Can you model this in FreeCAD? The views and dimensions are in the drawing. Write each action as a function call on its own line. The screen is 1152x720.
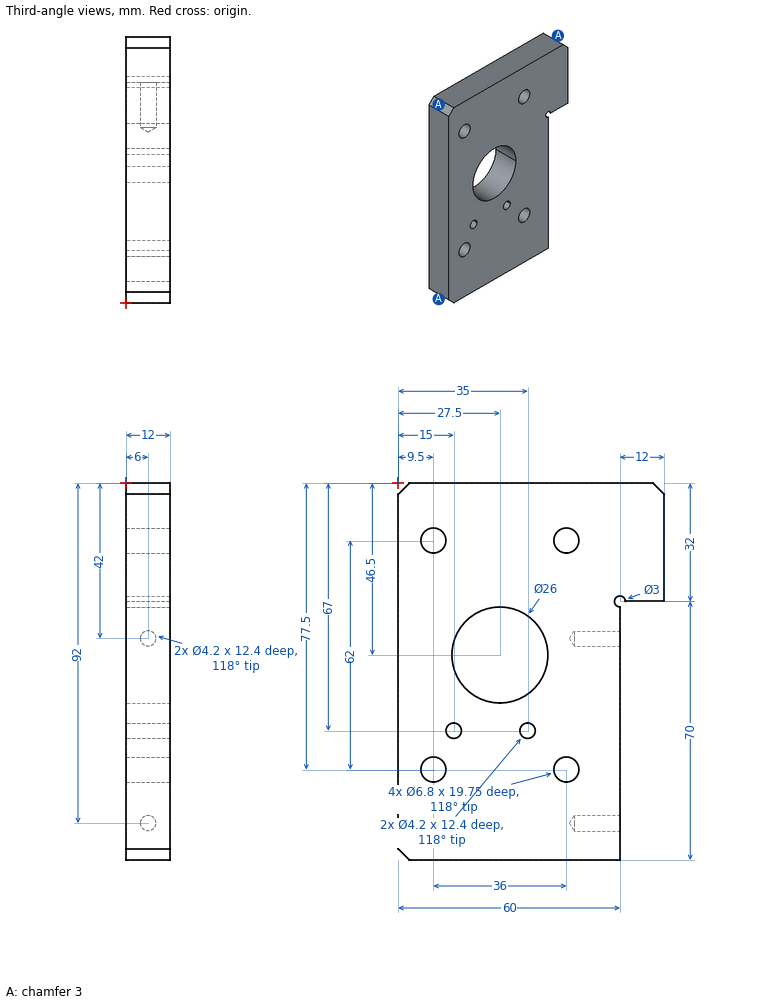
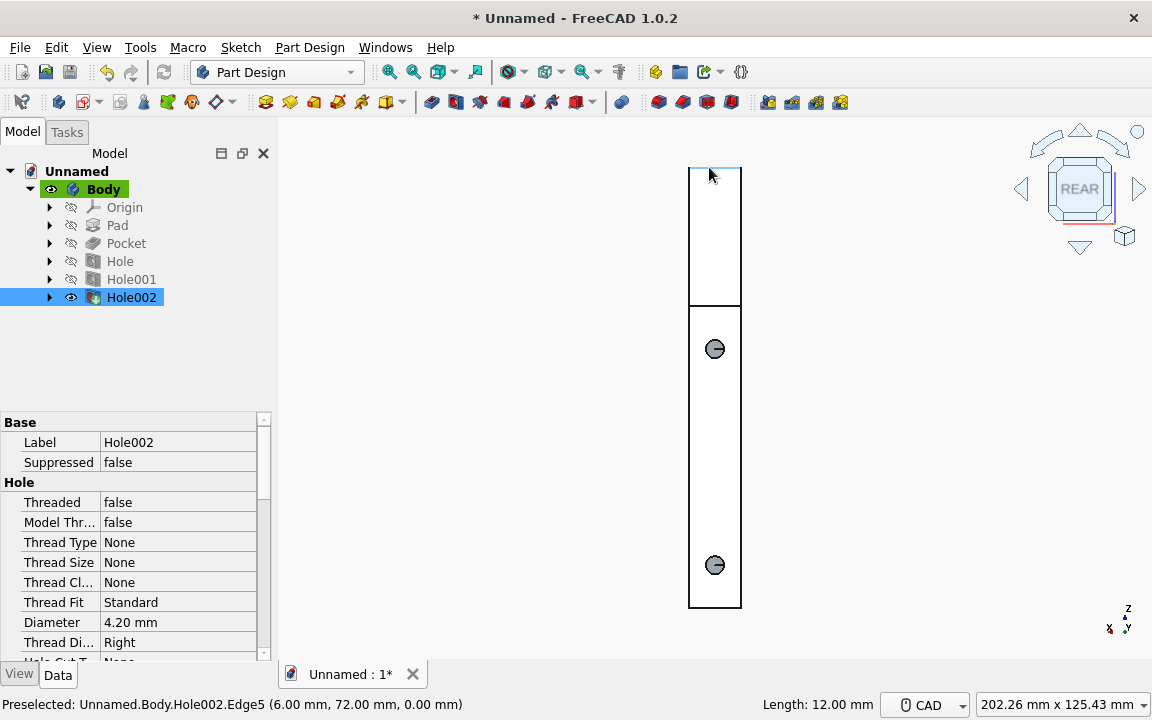
key(0)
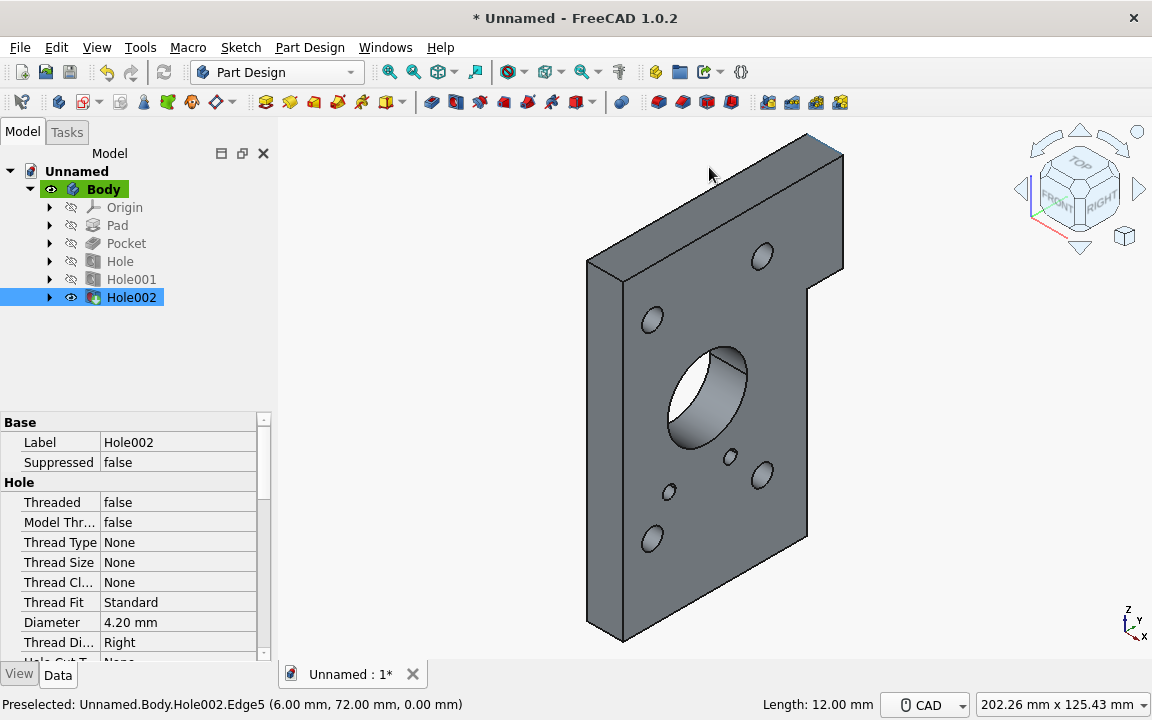
click(605, 271, ctrl)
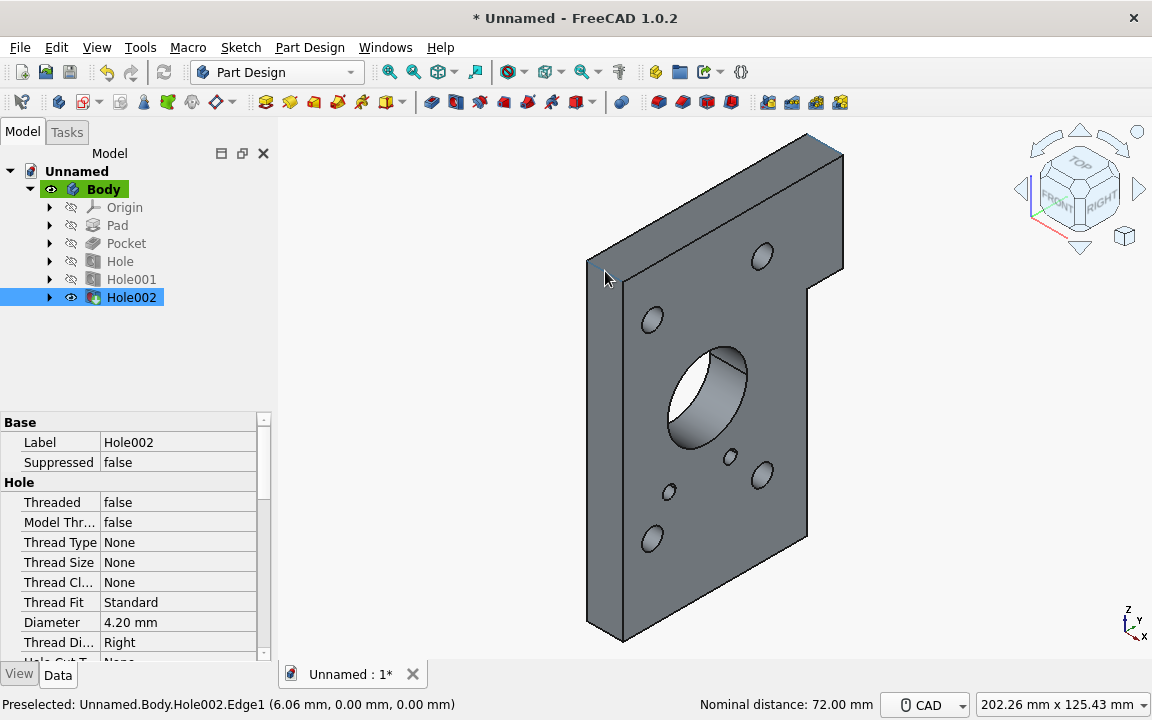
key(2)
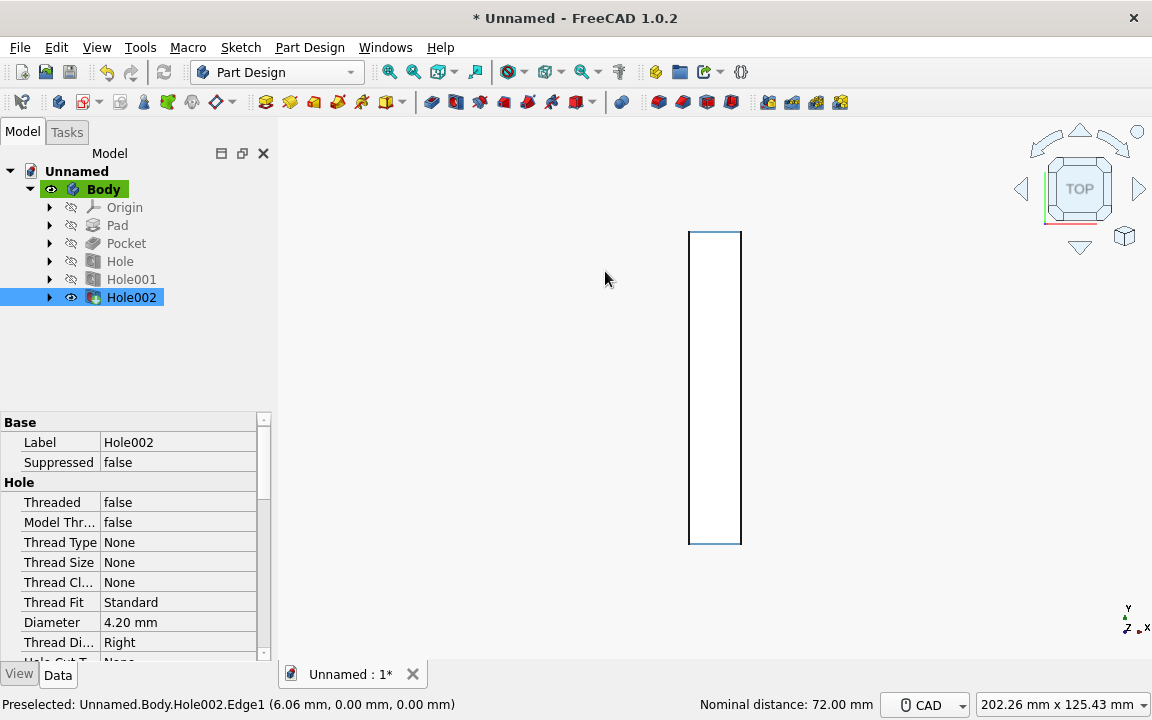
key(1)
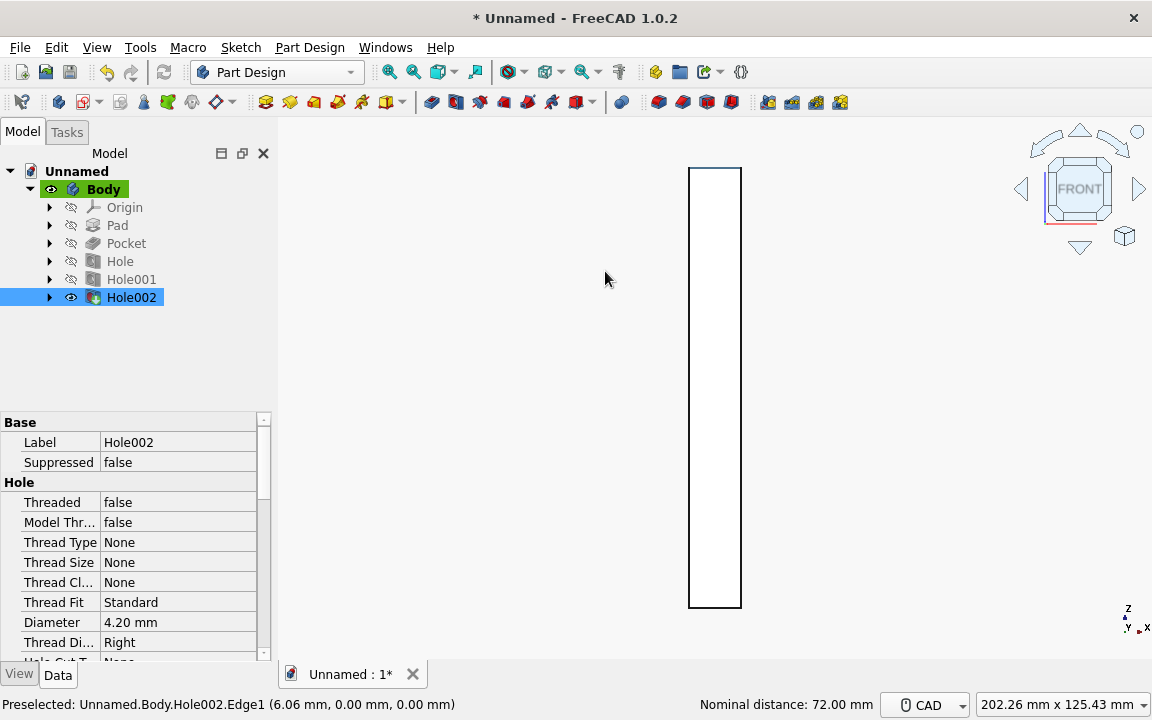
click(715, 607, ctrl)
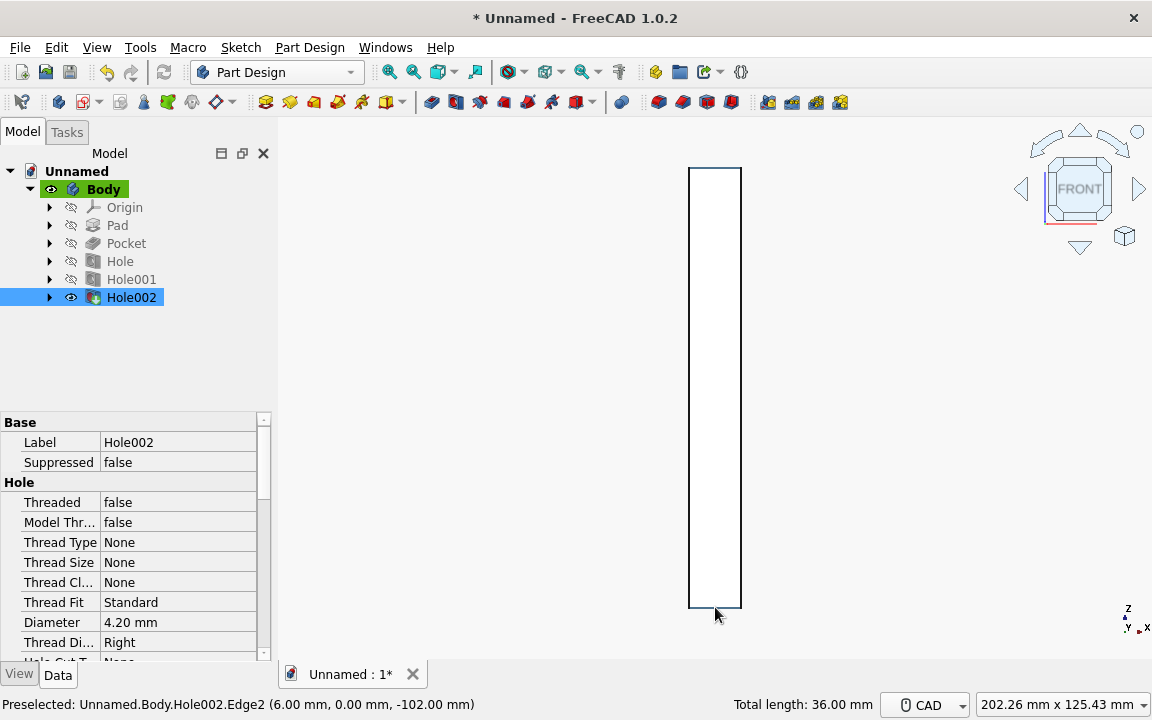
click(684, 102)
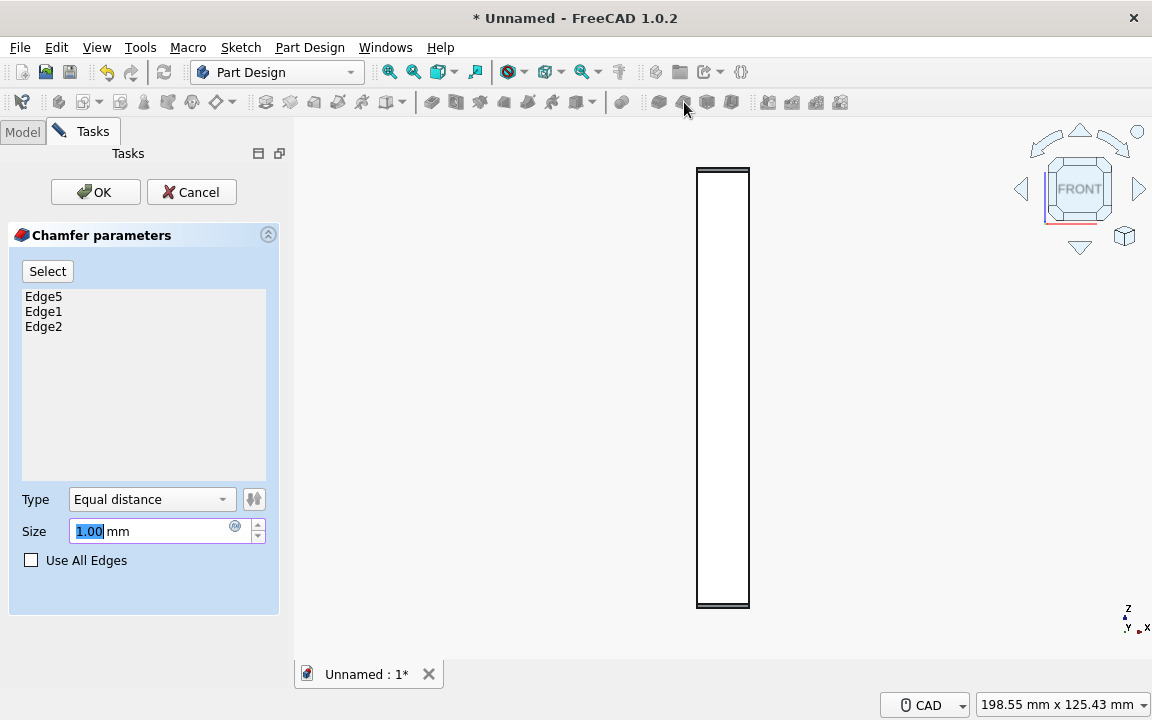
text(3)
key(Tab)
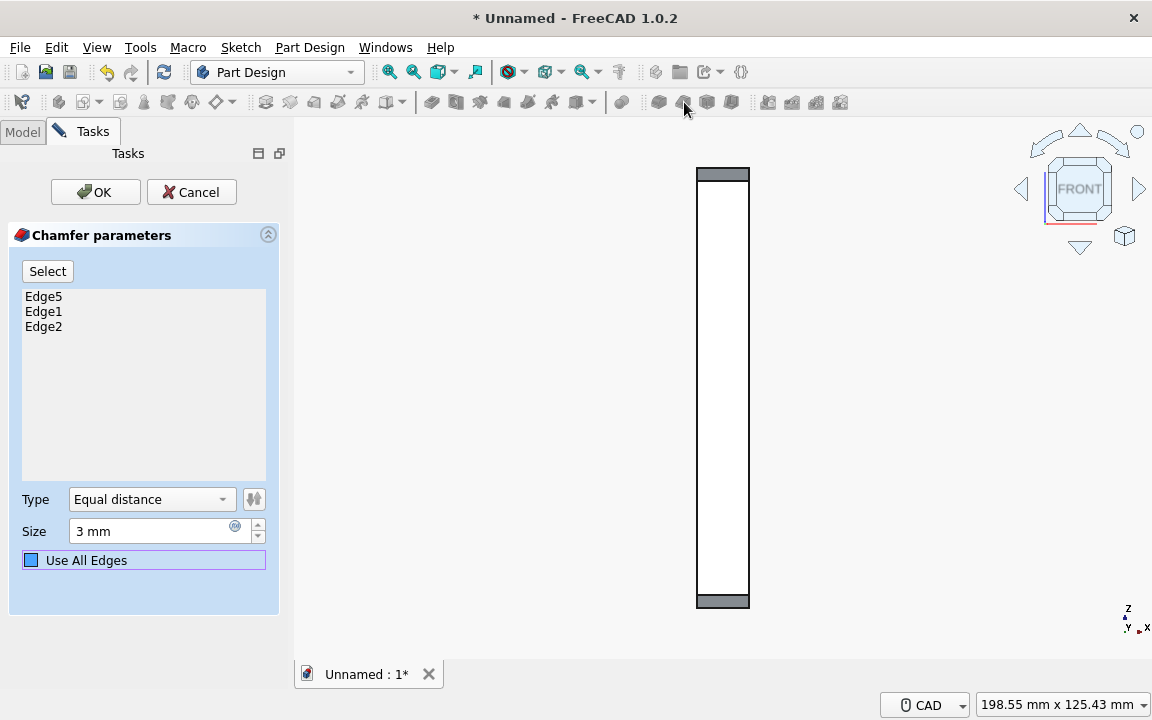
click(96, 192)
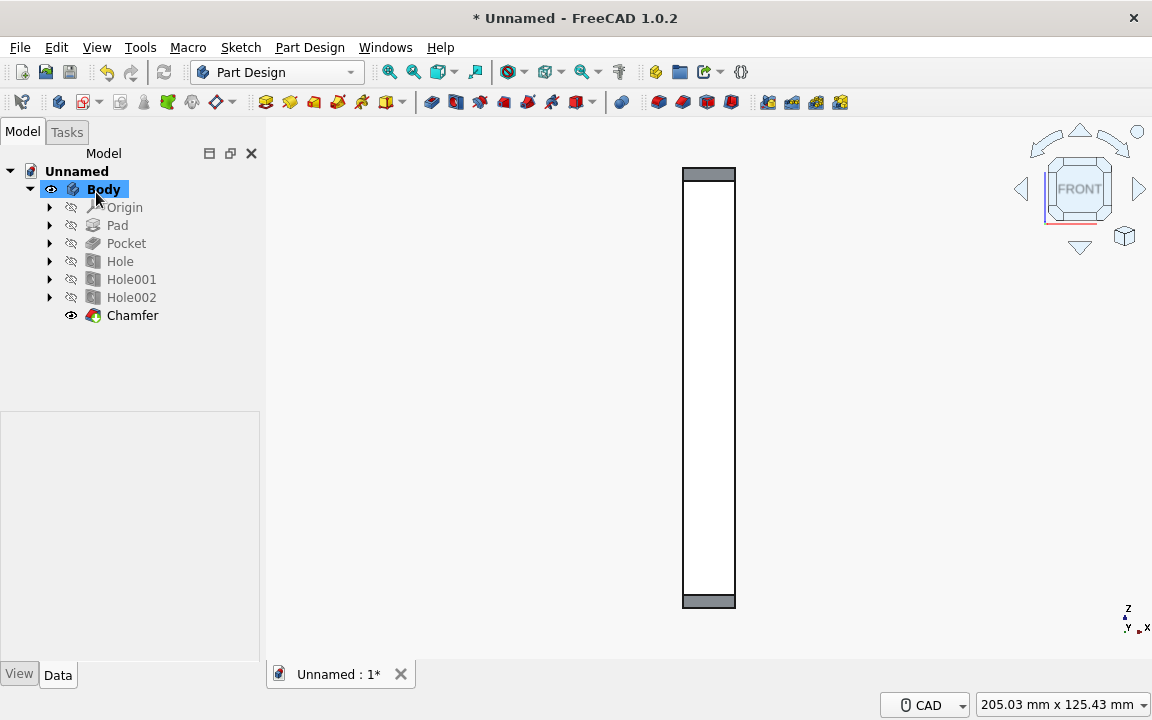
key(0)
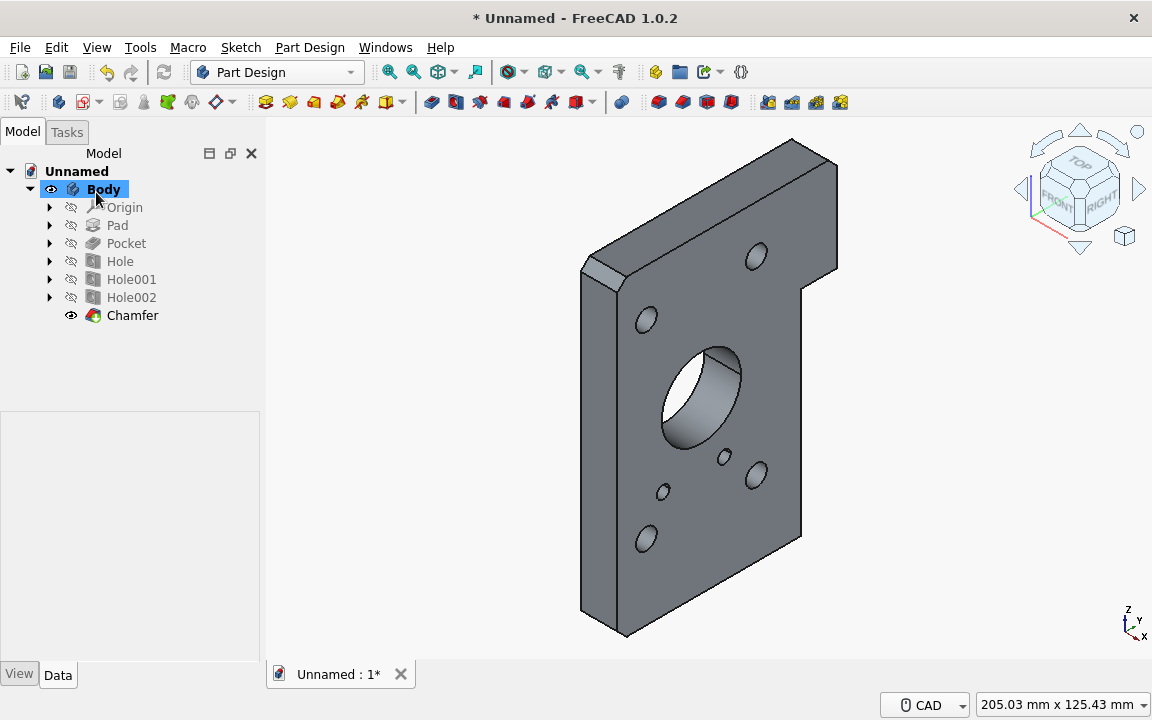
click(696, 519)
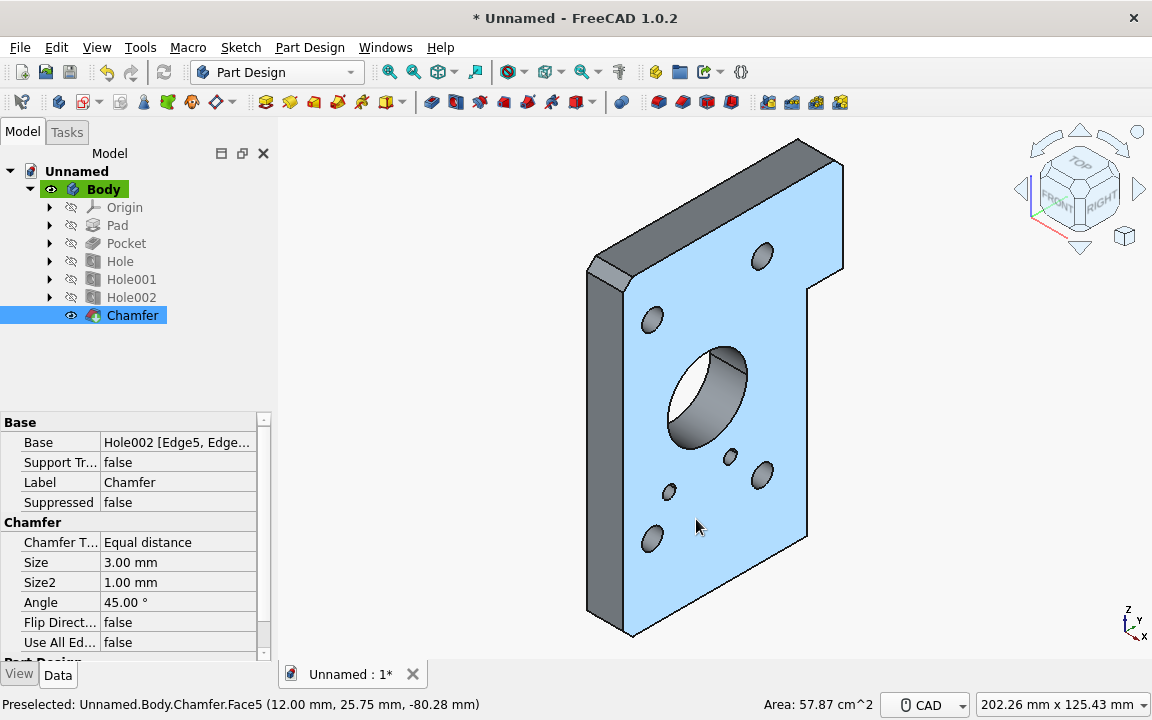
click(84, 102)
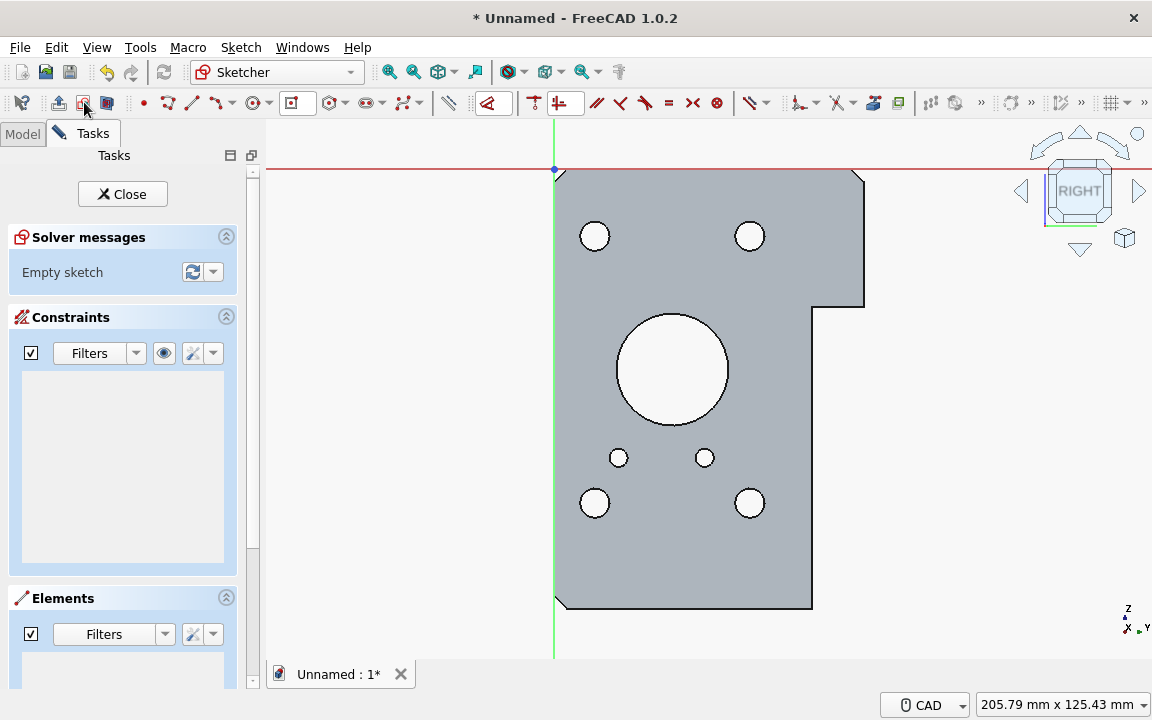
scroll(821, 303, up, 15)